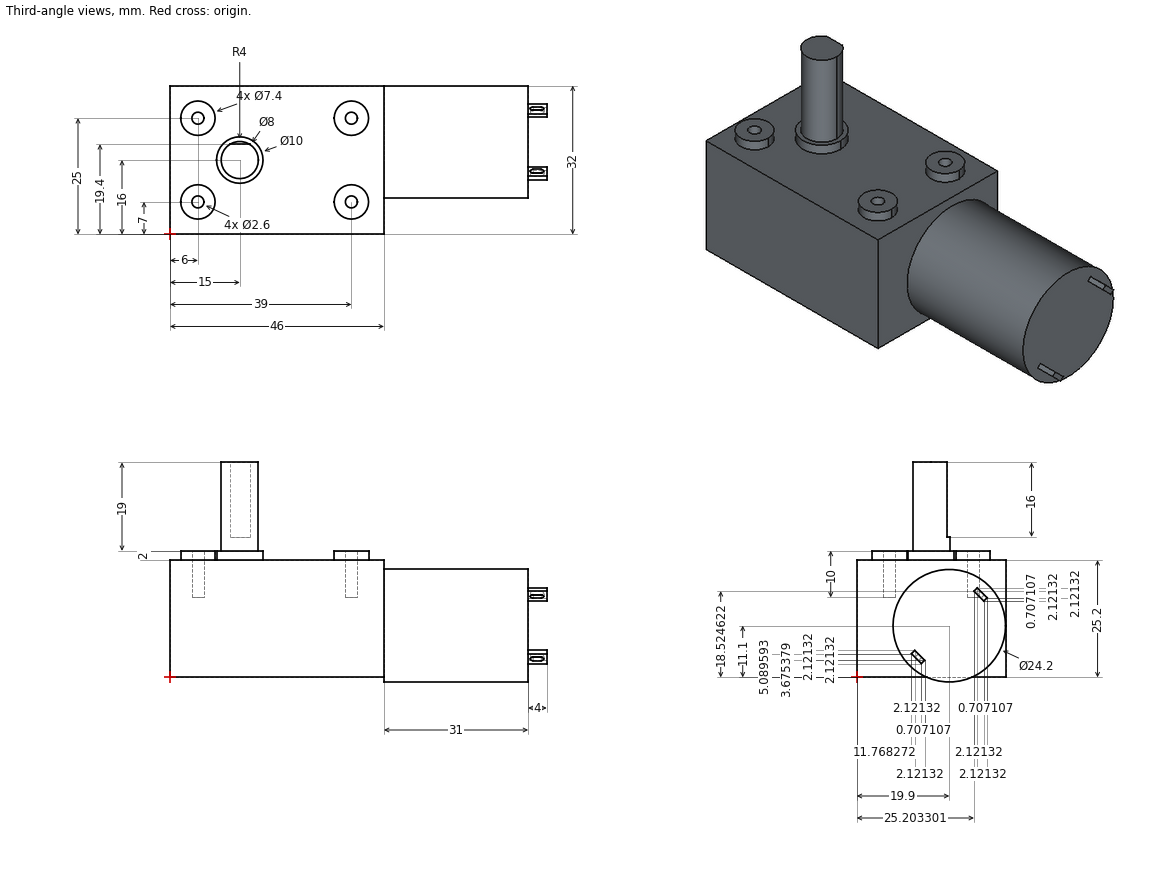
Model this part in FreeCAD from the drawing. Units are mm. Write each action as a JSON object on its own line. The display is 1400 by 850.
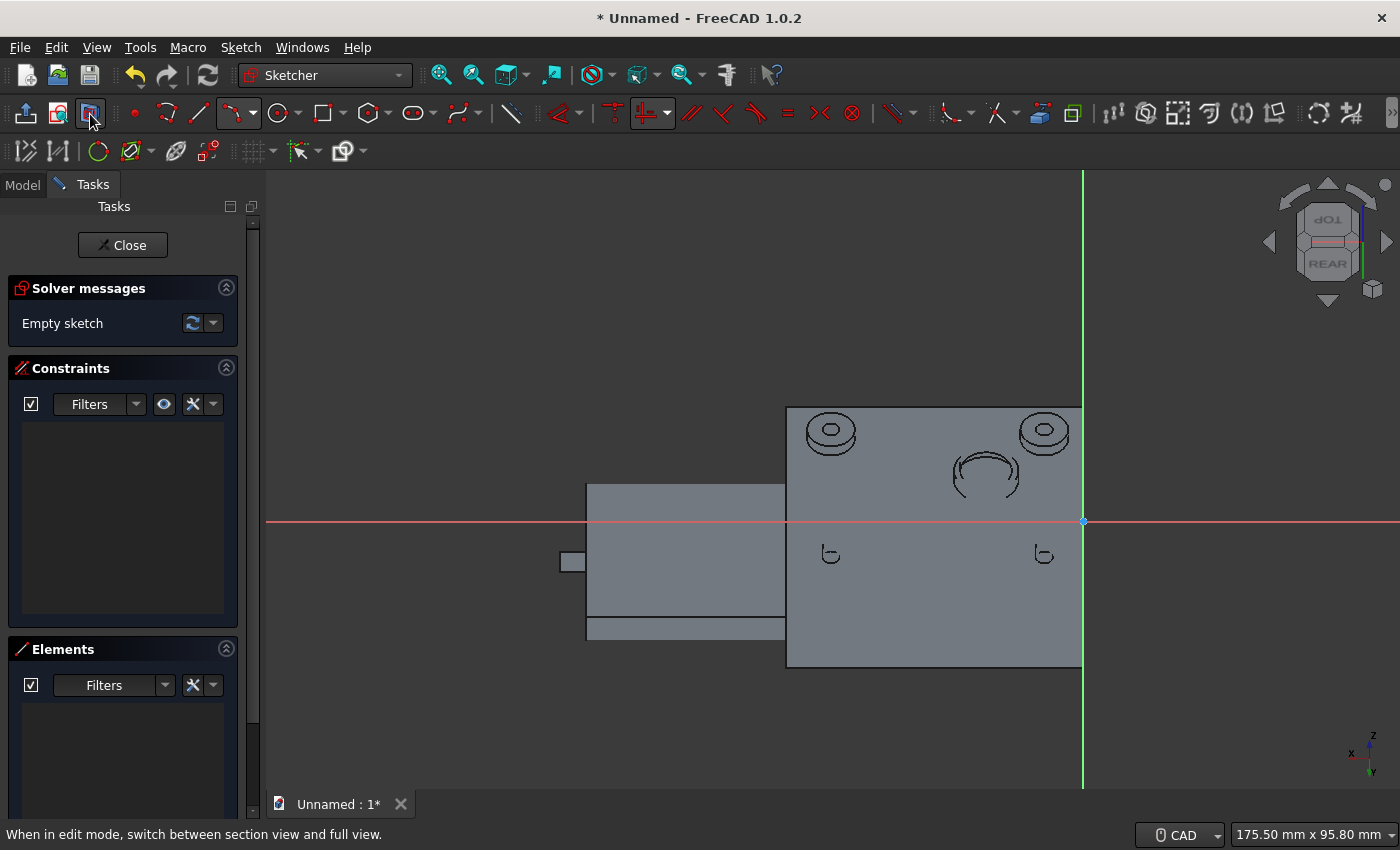
{"action": "scroll", "coordinate": [563, 567], "scroll_direction": "up", "scroll_amount": 15}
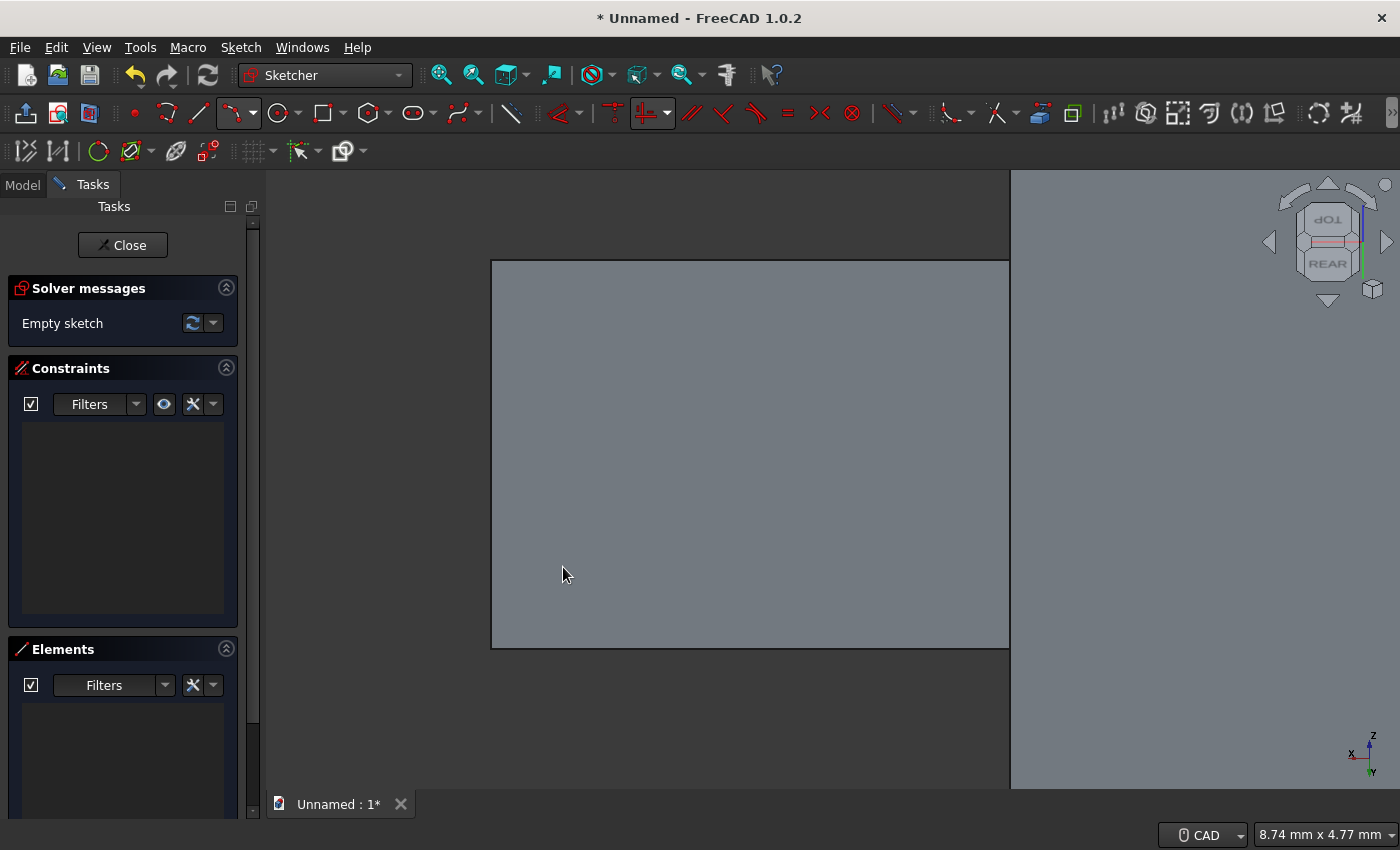
{"action": "scroll", "coordinate": [764, 453], "scroll_direction": "up", "scroll_amount": 3}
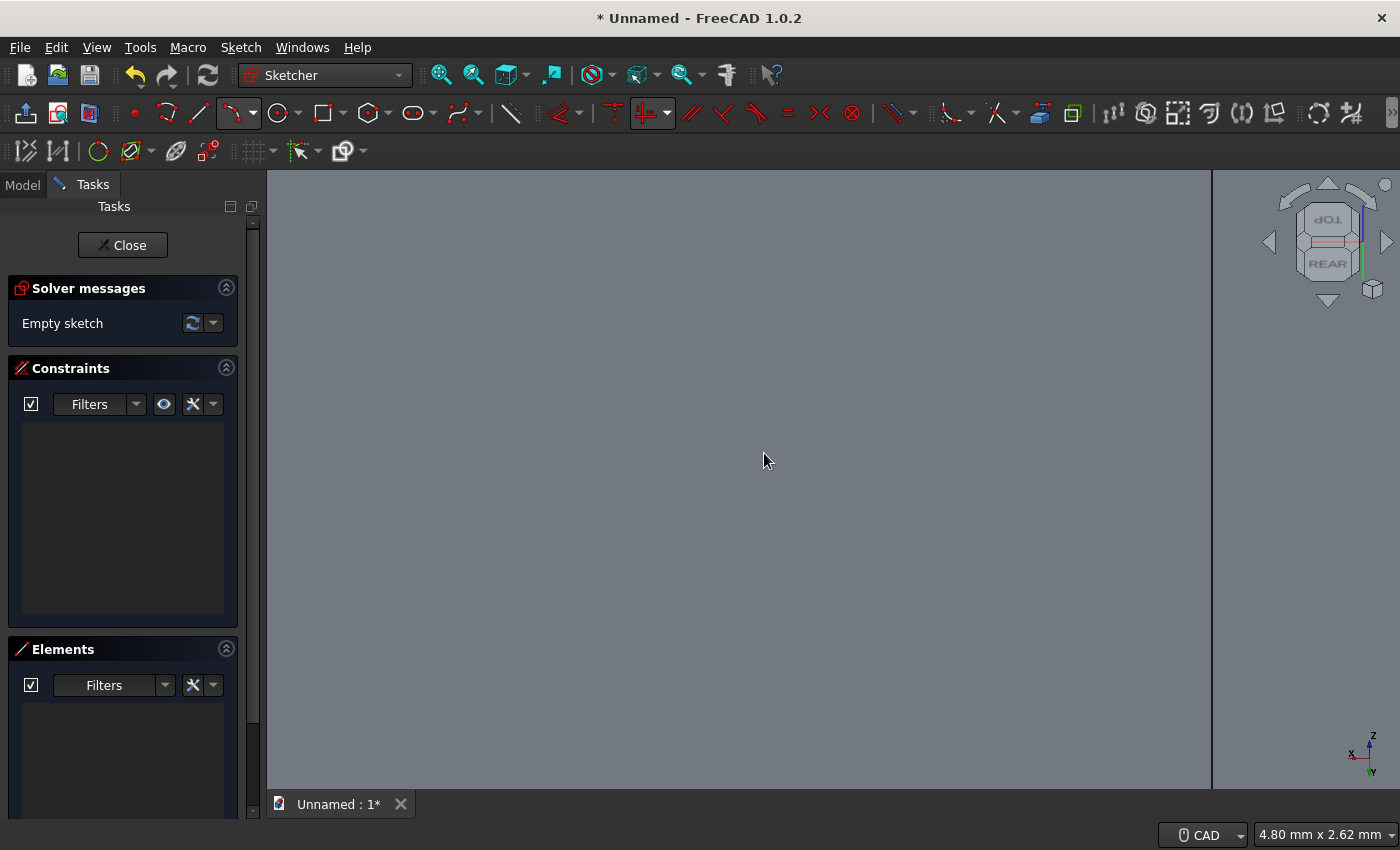
{"action": "key", "text": "g s"}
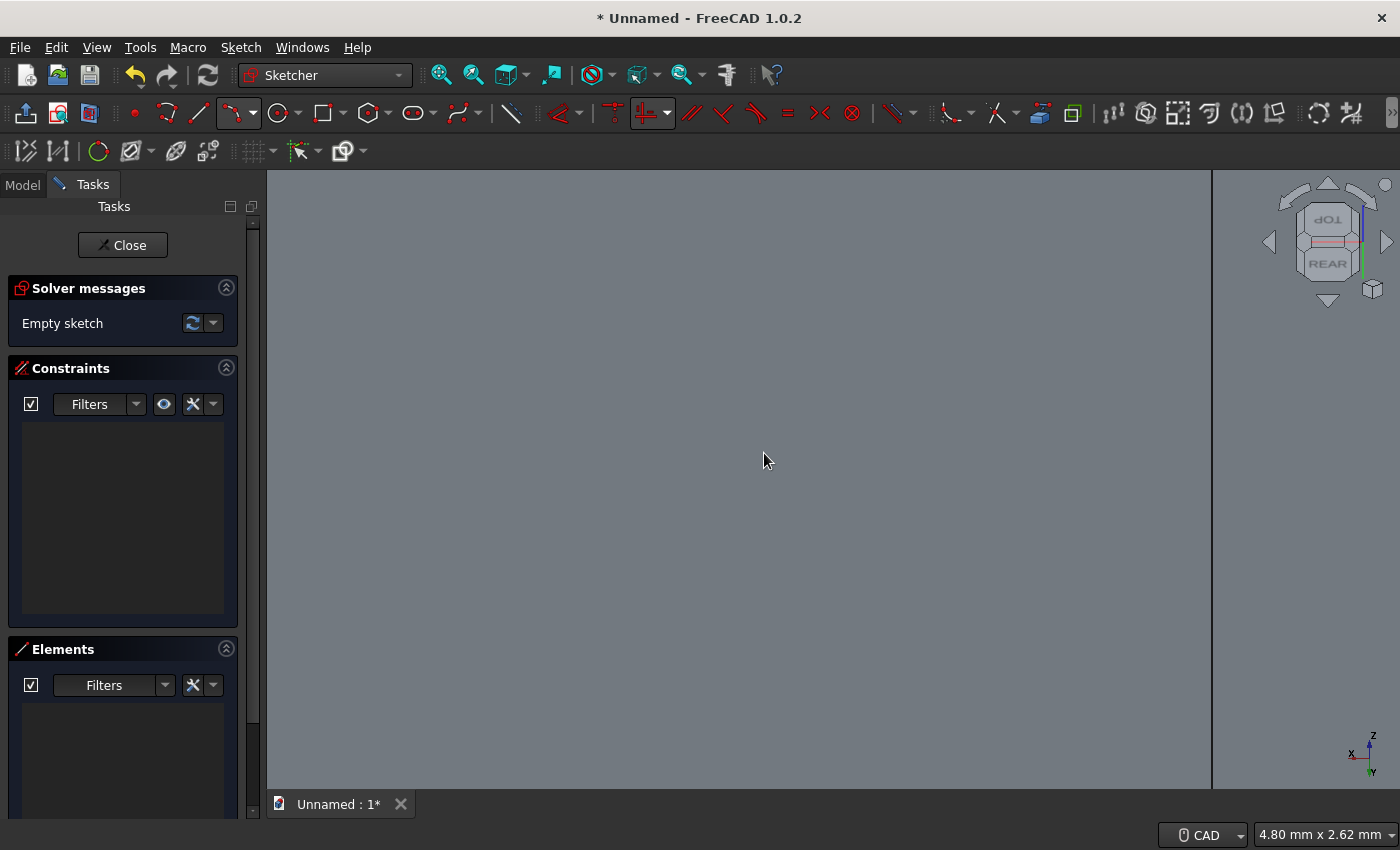
{"action": "left_click", "coordinate": [545, 479]}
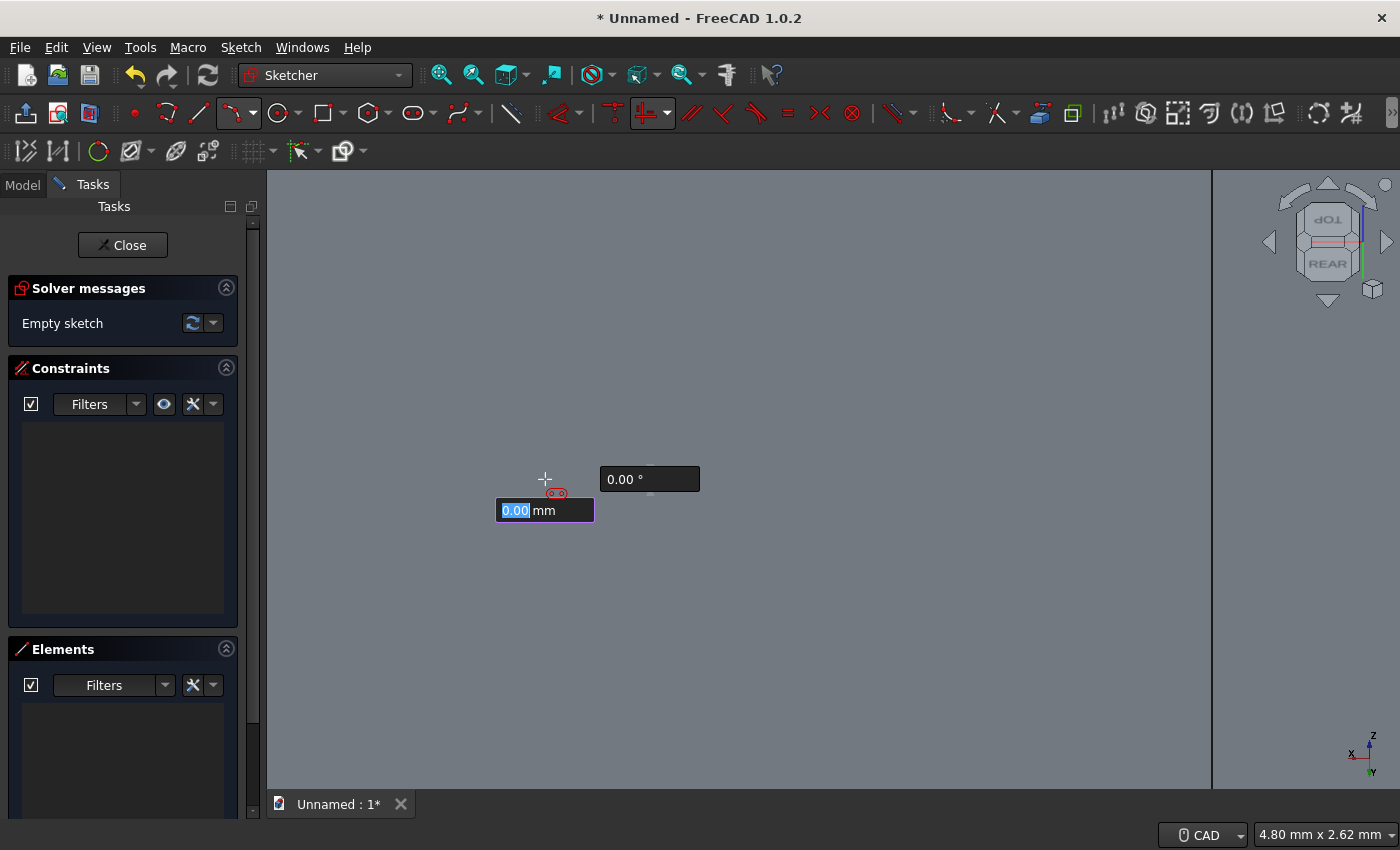
{"action": "left_click", "coordinate": [983, 479]}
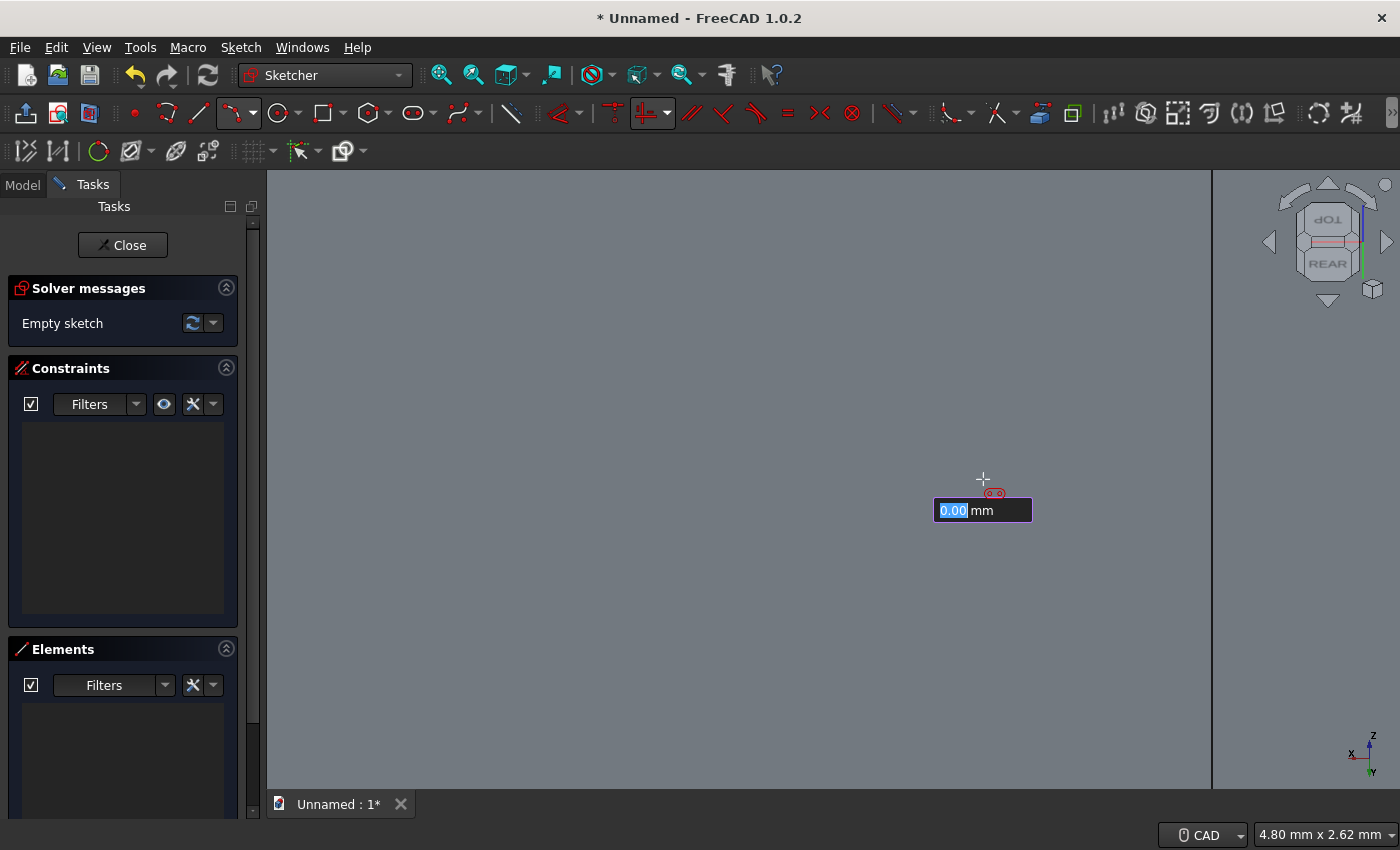
{"action": "left_click", "coordinate": [764, 602]}
{"action": "key", "text": "Escape"}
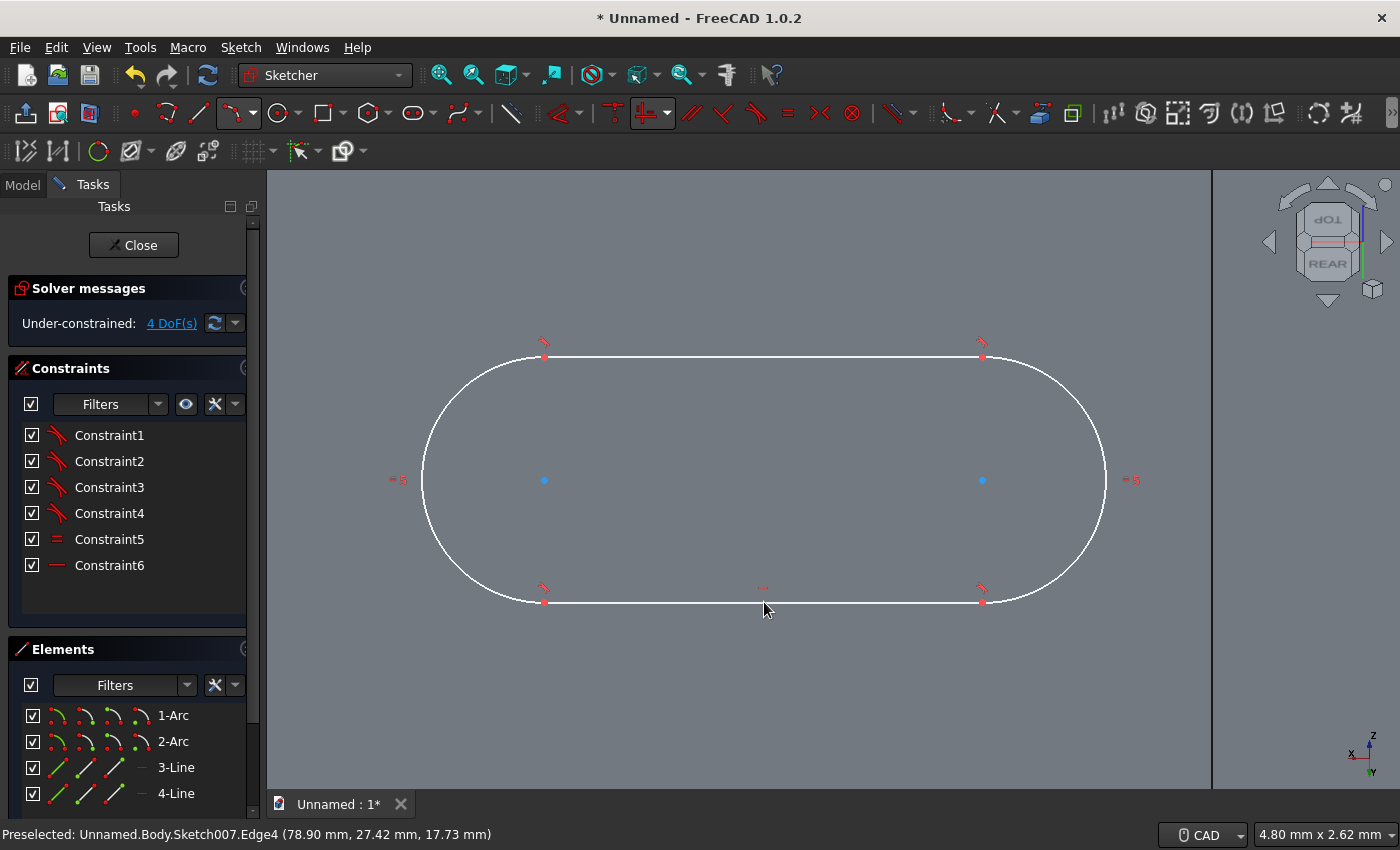
{"action": "left_click", "coordinate": [558, 114]}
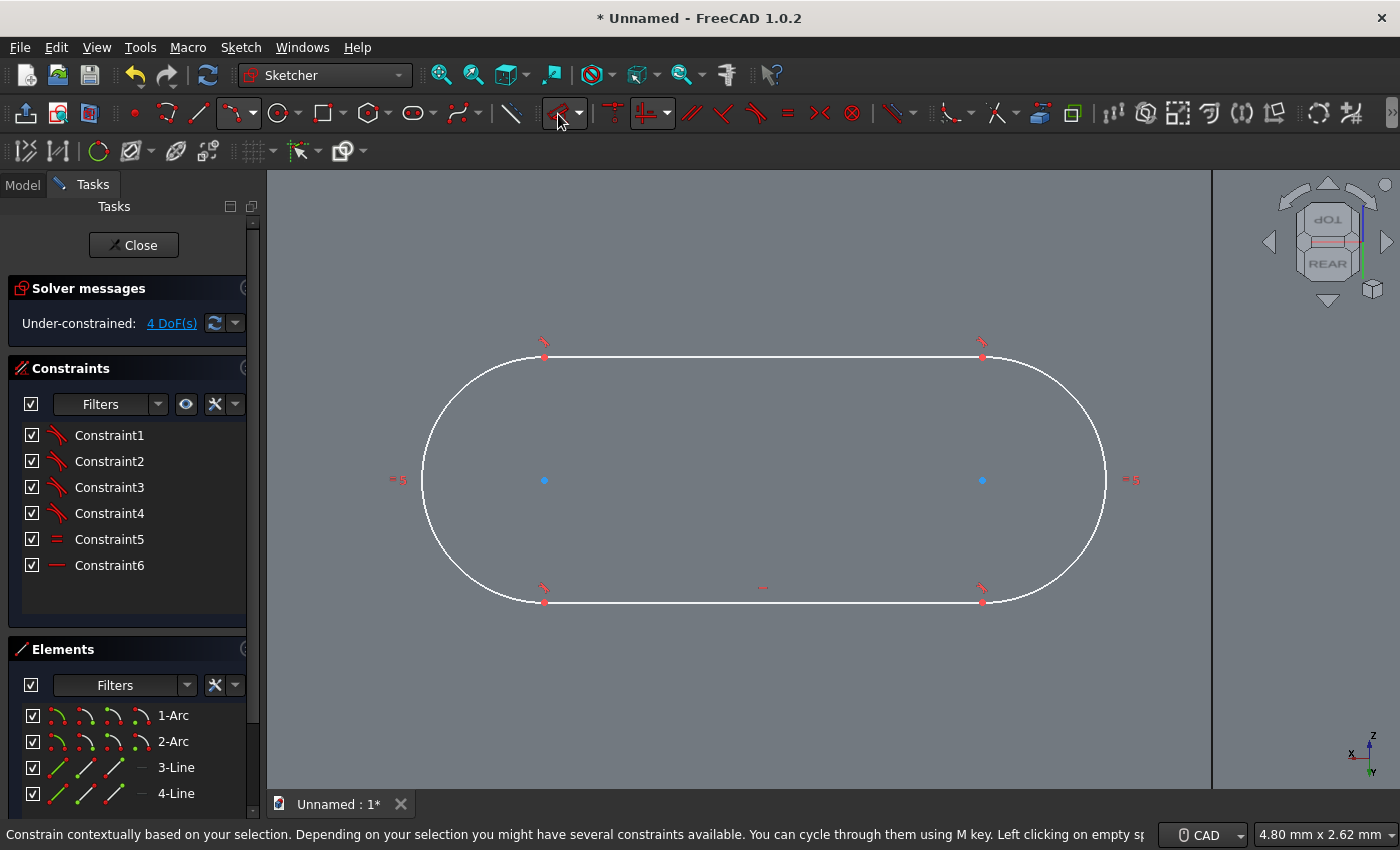
{"action": "left_click", "coordinate": [445, 408]}
{"action": "left_click", "coordinate": [419, 389]}